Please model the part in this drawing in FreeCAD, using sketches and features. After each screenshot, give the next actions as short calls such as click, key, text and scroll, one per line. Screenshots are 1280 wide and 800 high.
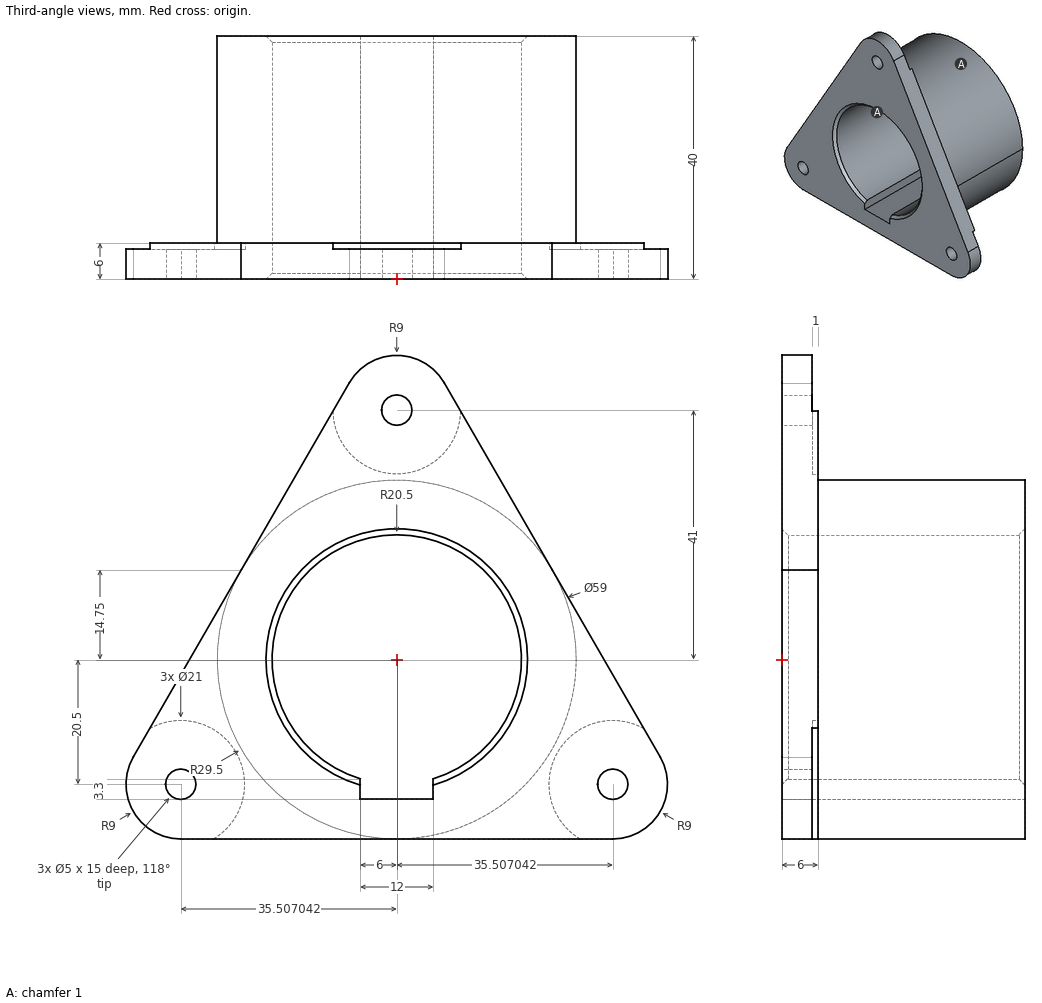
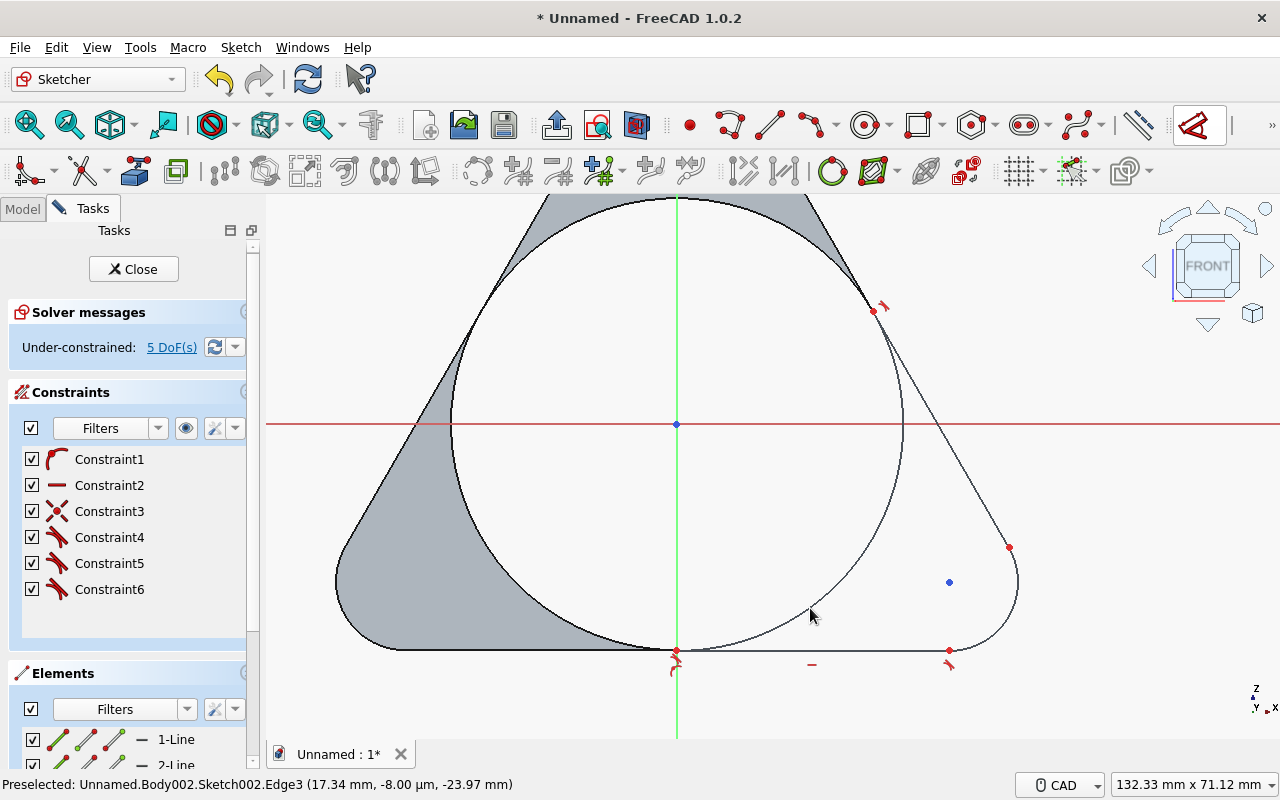
click(914, 383)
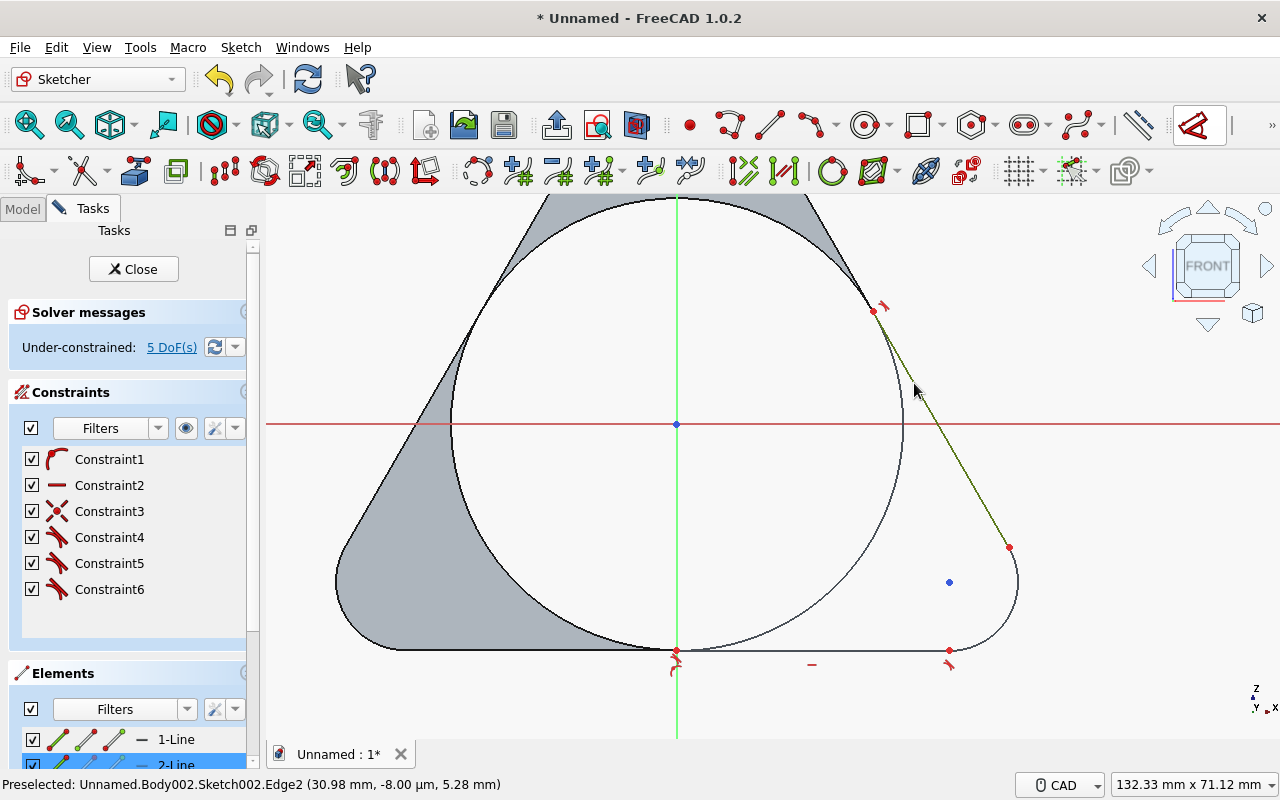
click(989, 638)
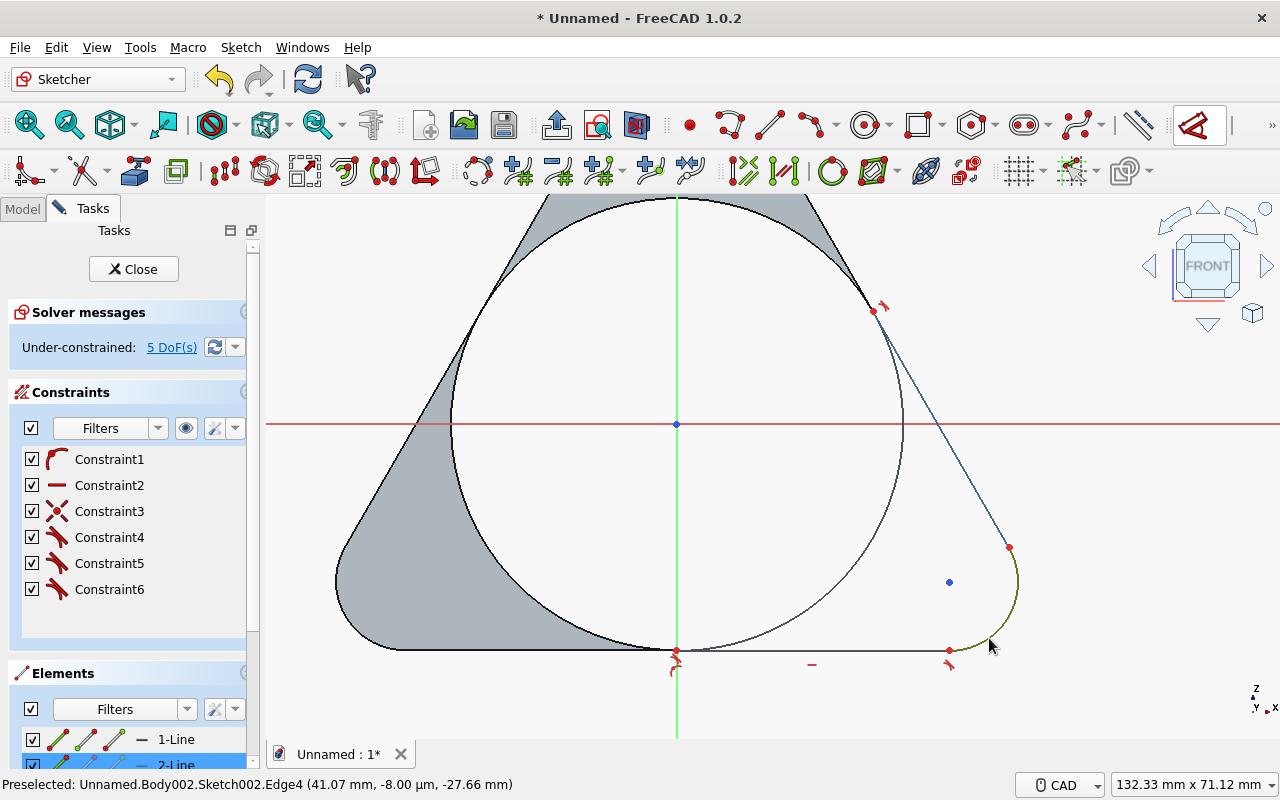
key(t)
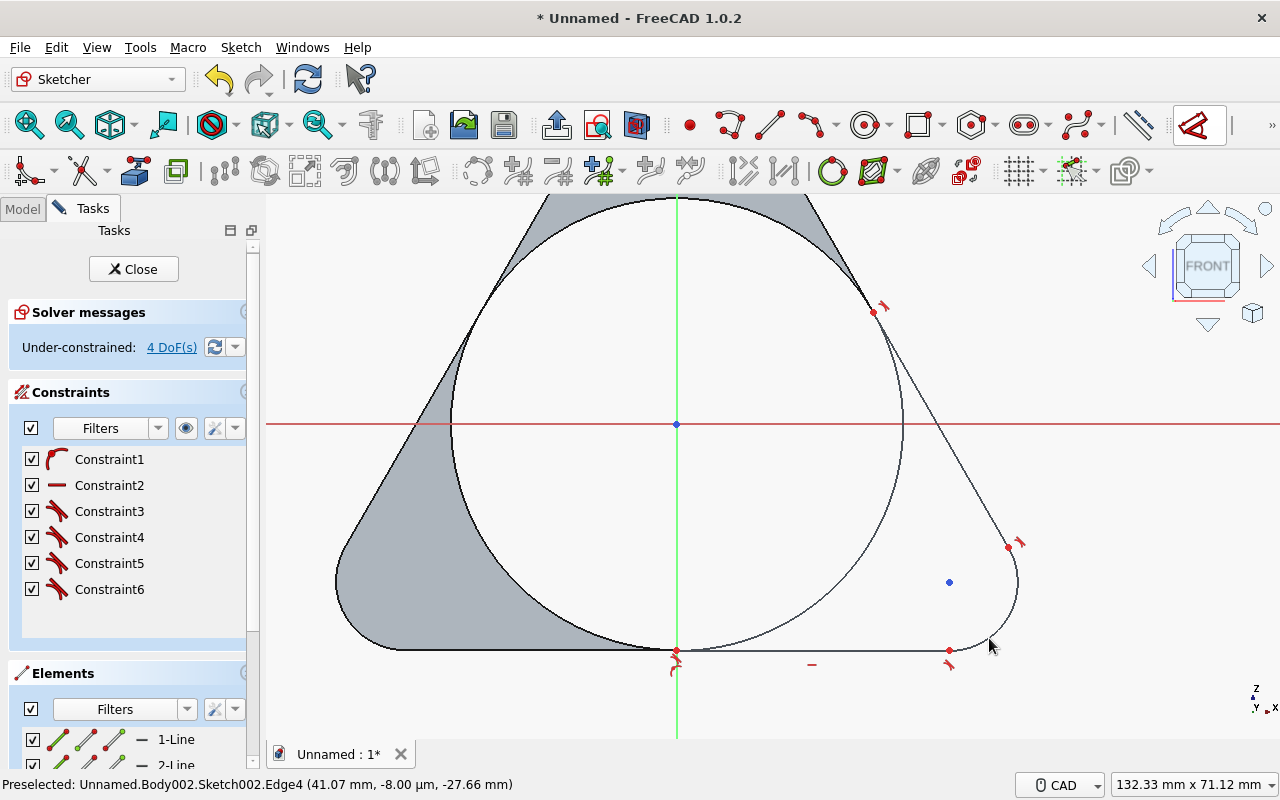
click(677, 425)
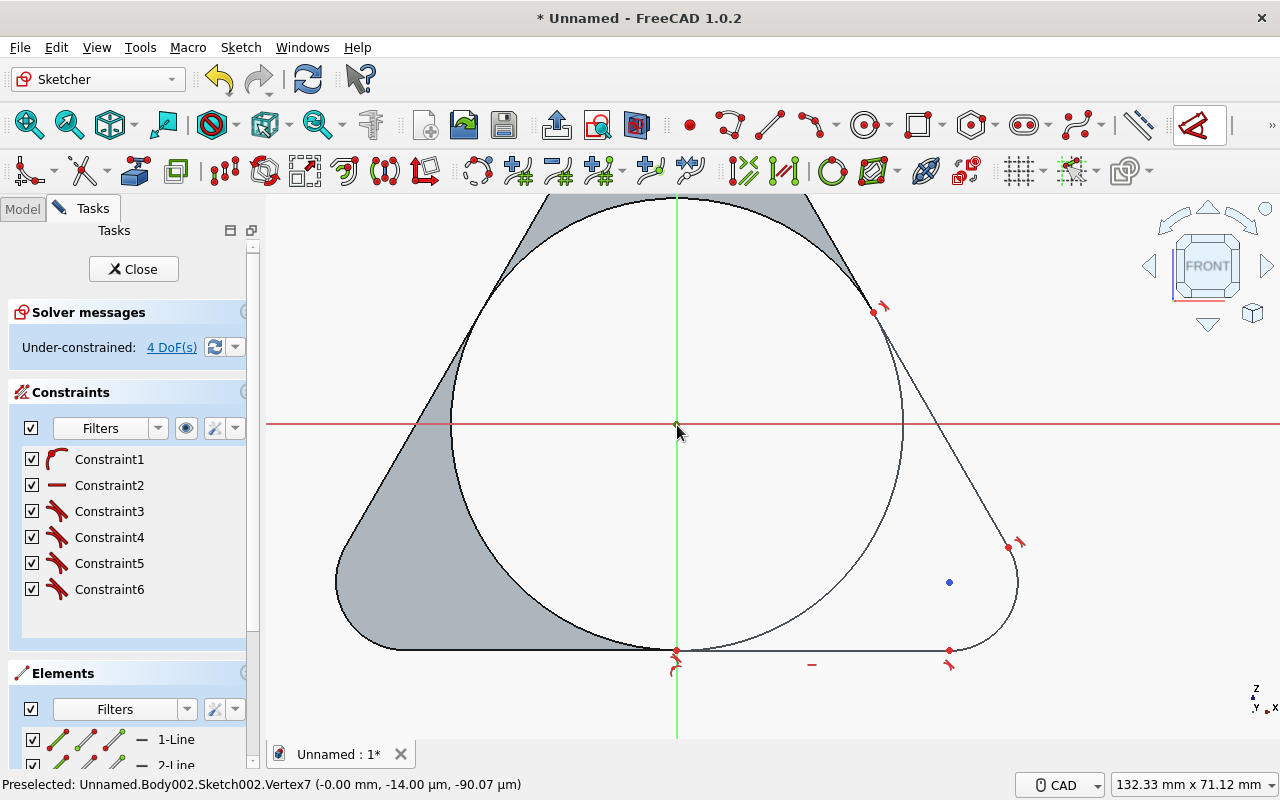
click(353, 424)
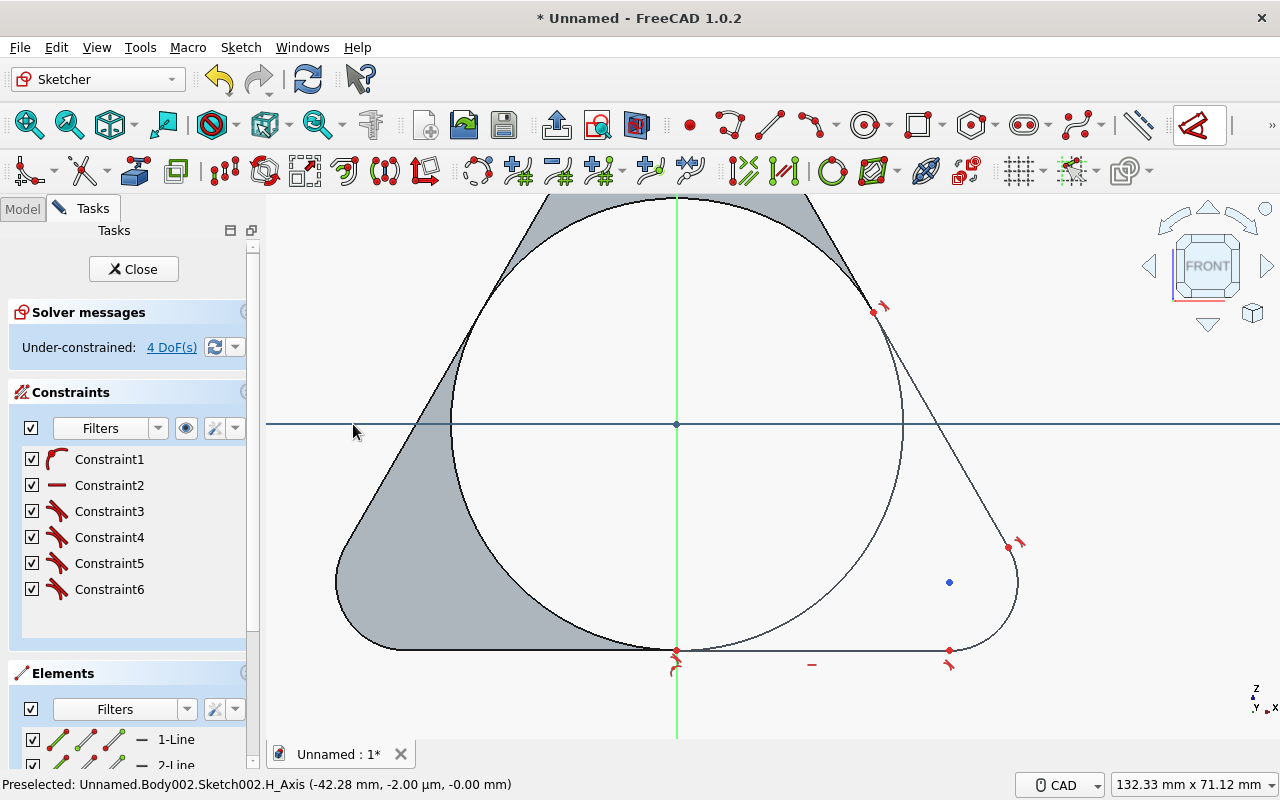
key(c)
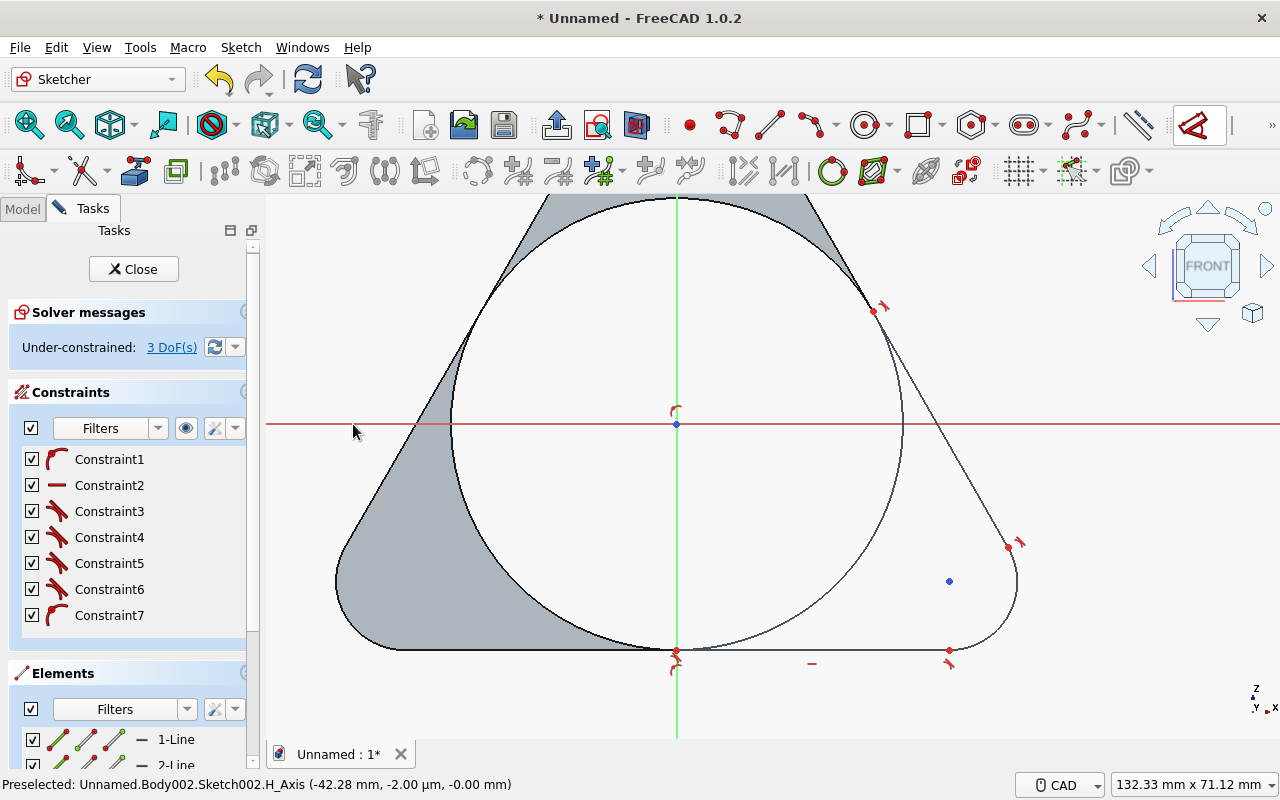
click(810, 607)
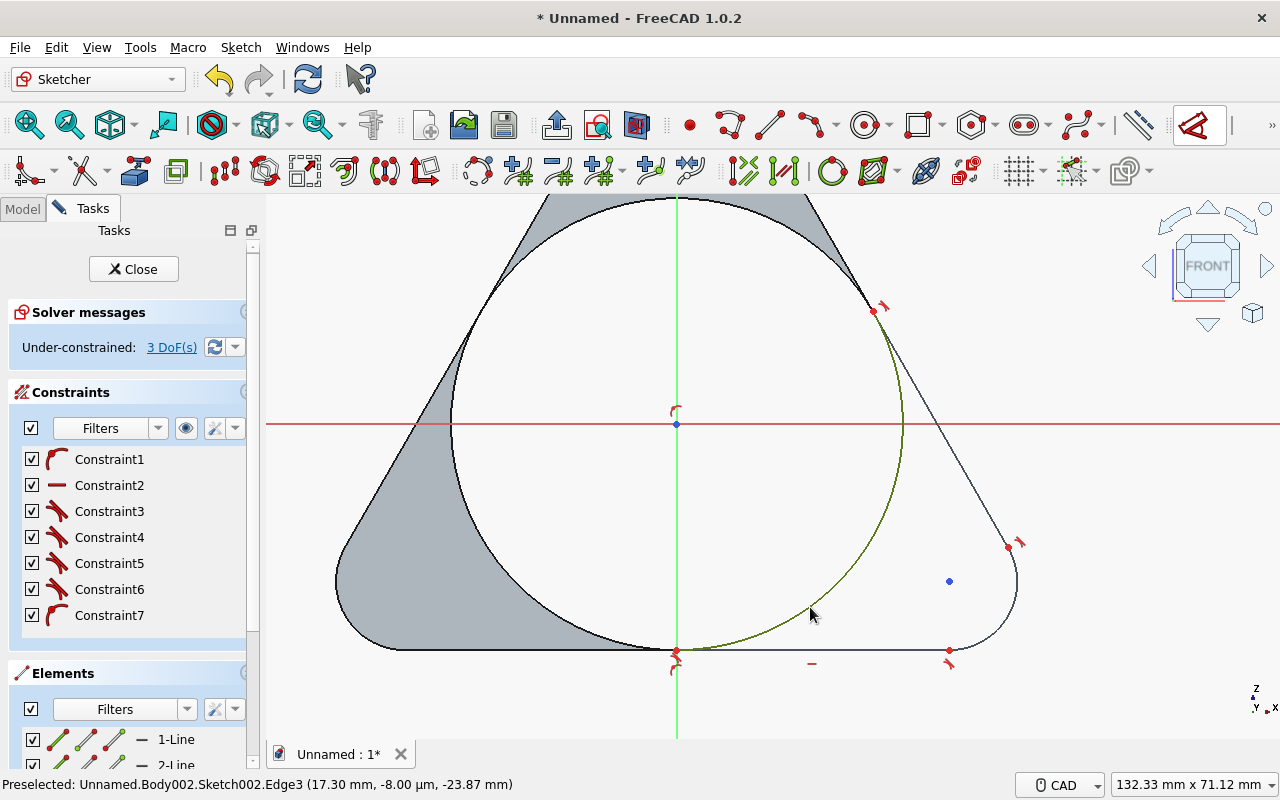
key(k)
key(r)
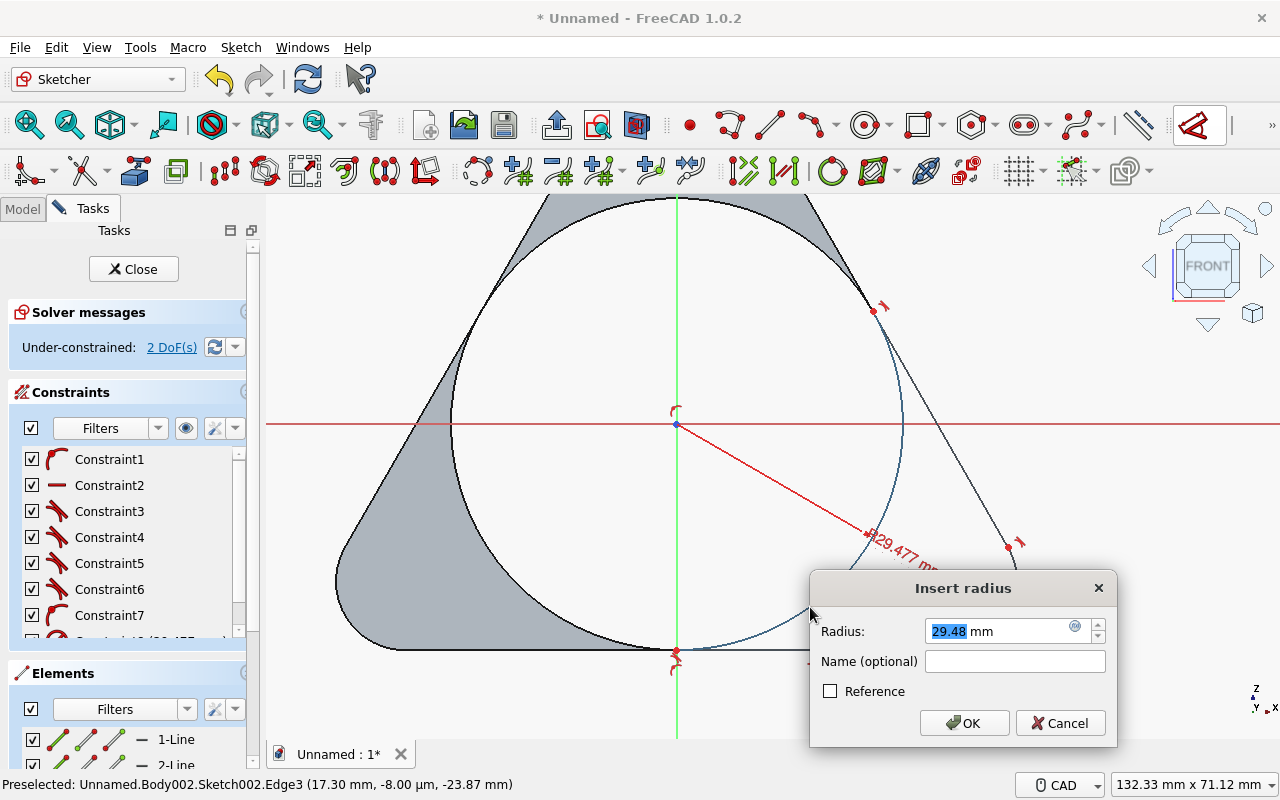
text(29.5)
key(Return)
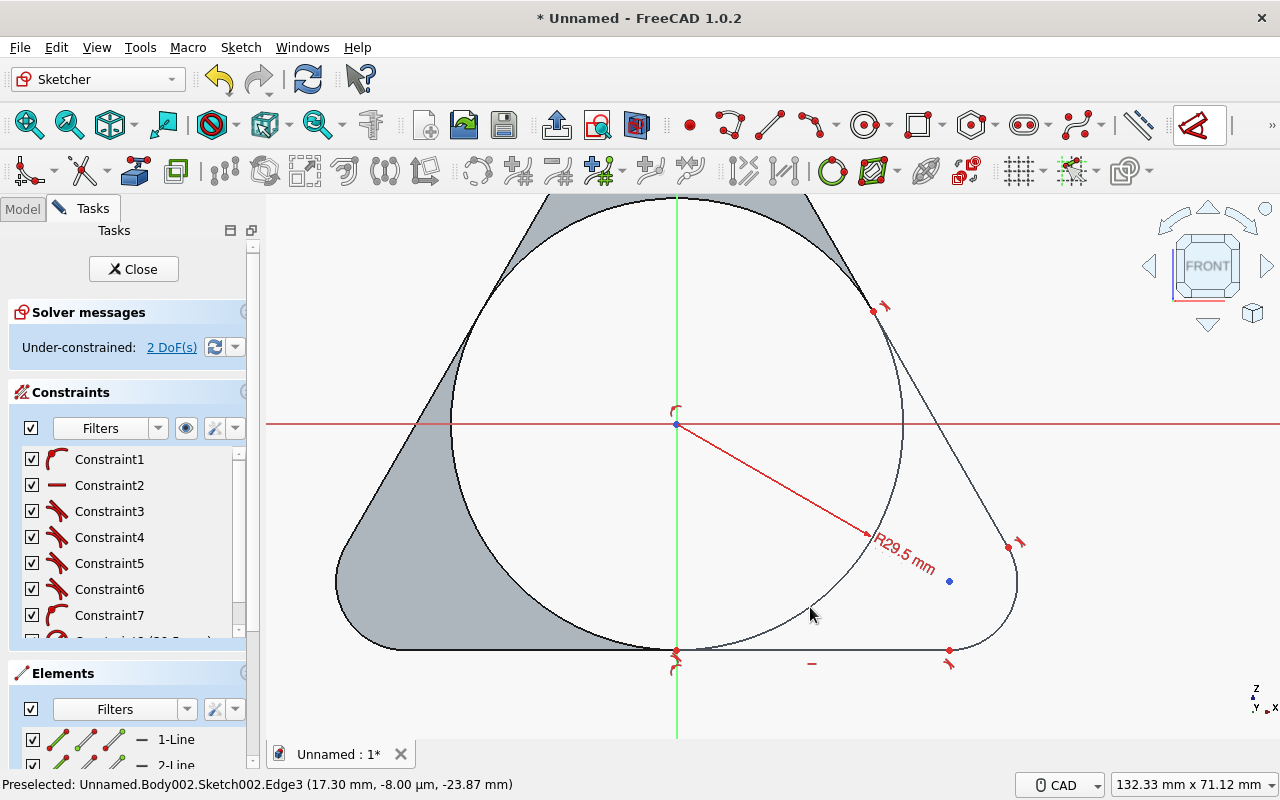
click(989, 637)